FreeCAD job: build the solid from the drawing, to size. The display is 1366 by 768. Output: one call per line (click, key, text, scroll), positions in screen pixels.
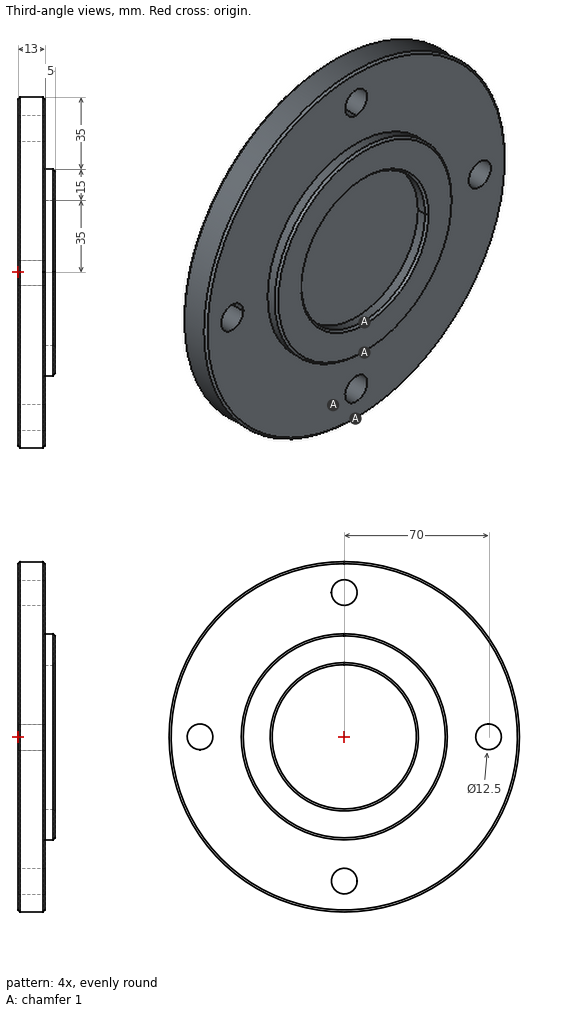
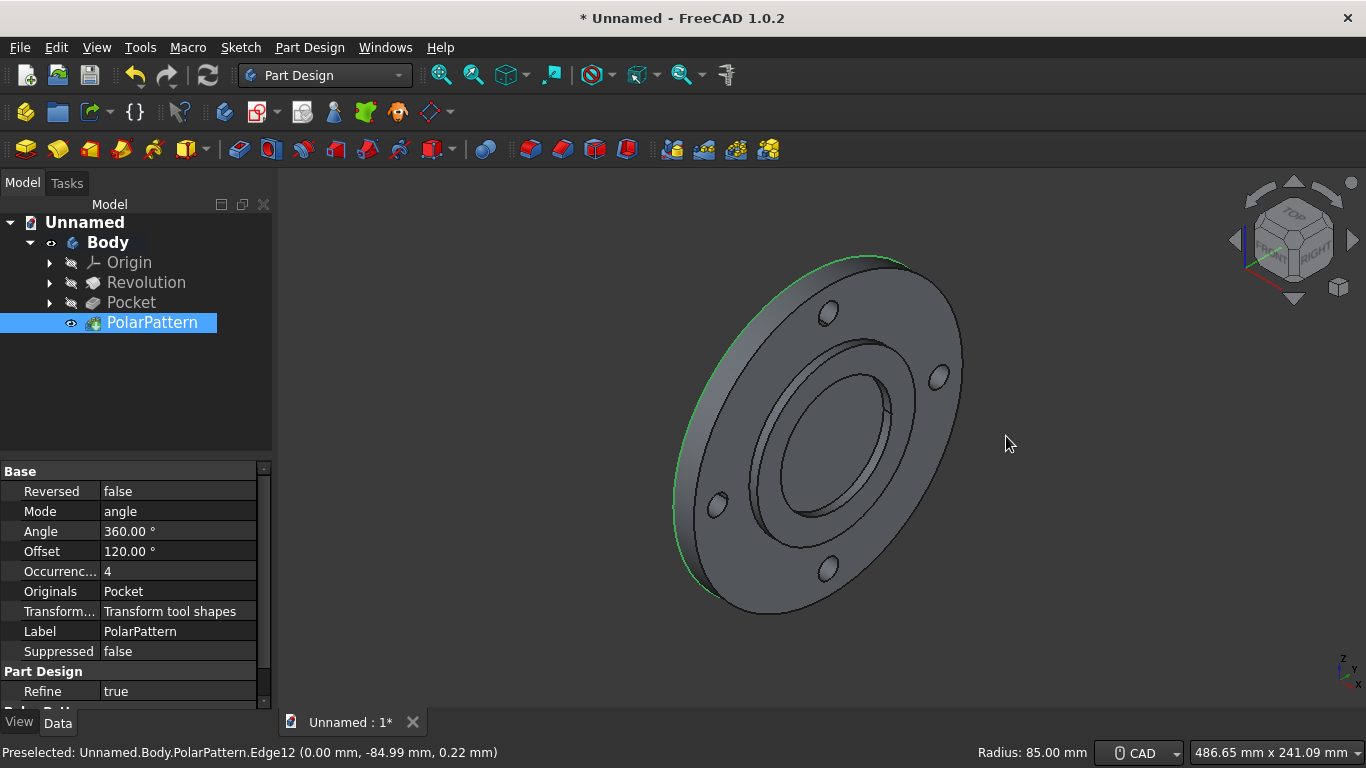
click(819, 515, ctrl)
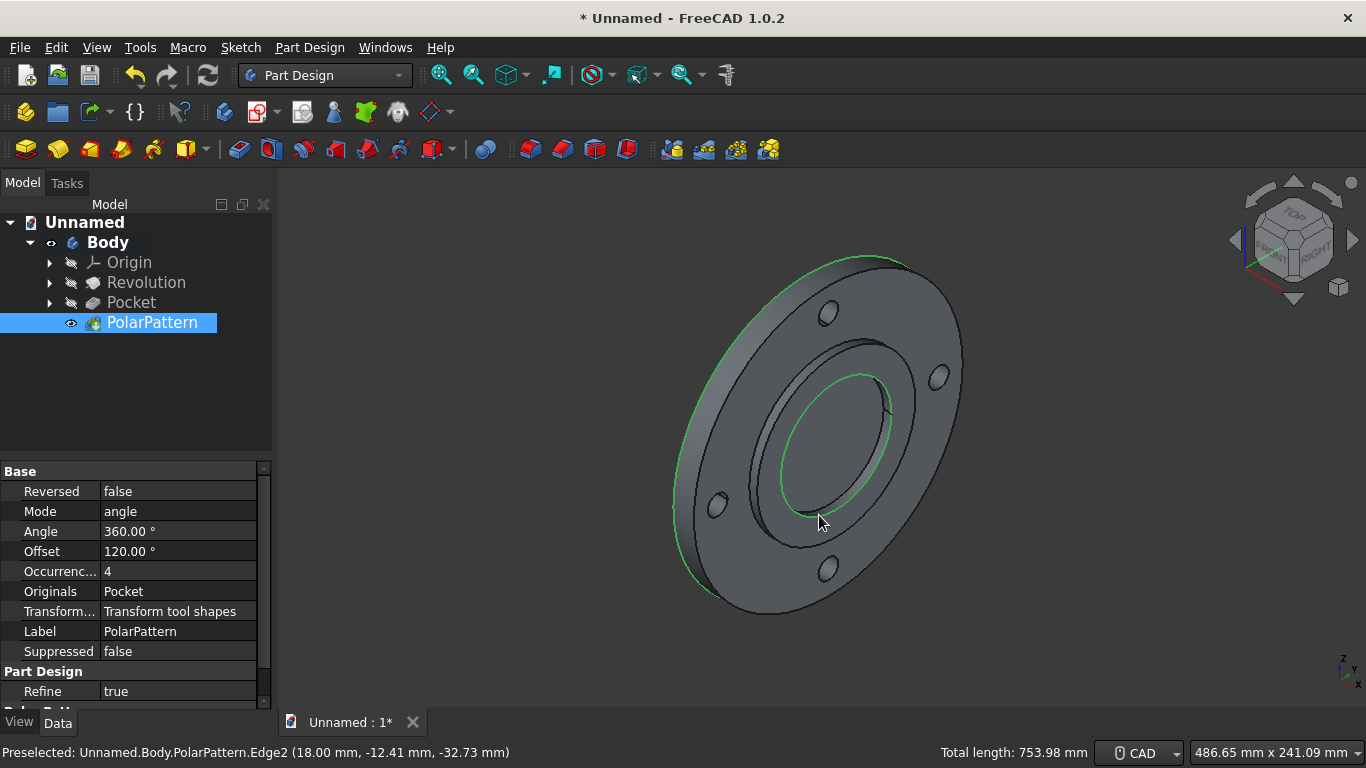
click(757, 490, ctrl)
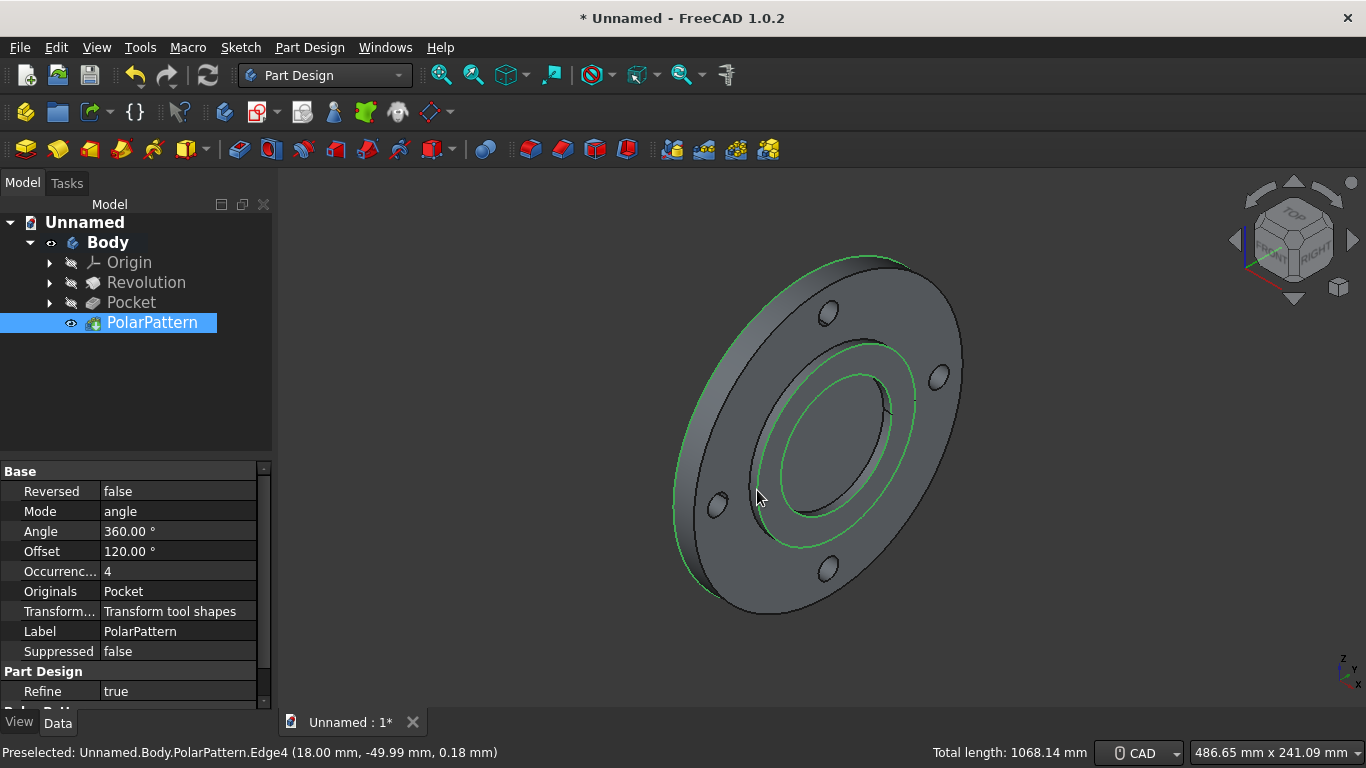
click(694, 518, ctrl)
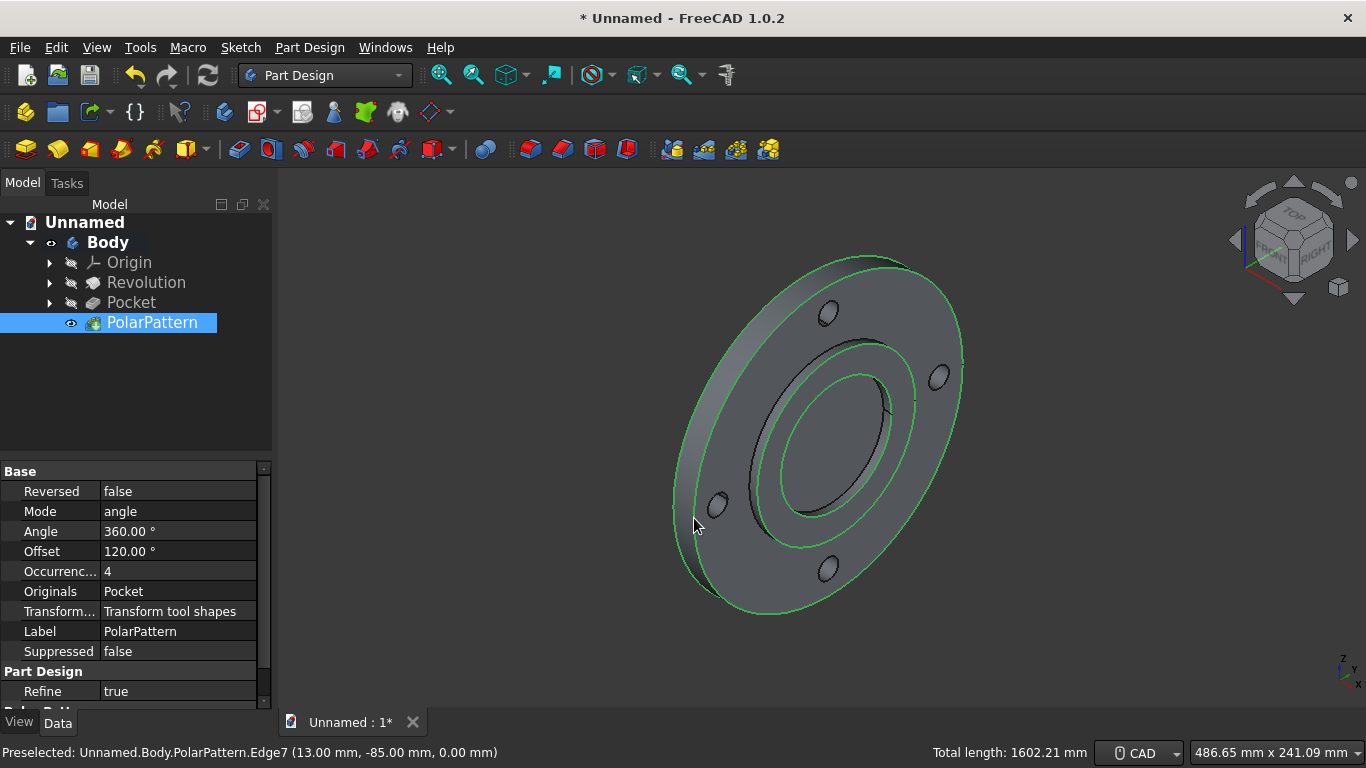
click(564, 150)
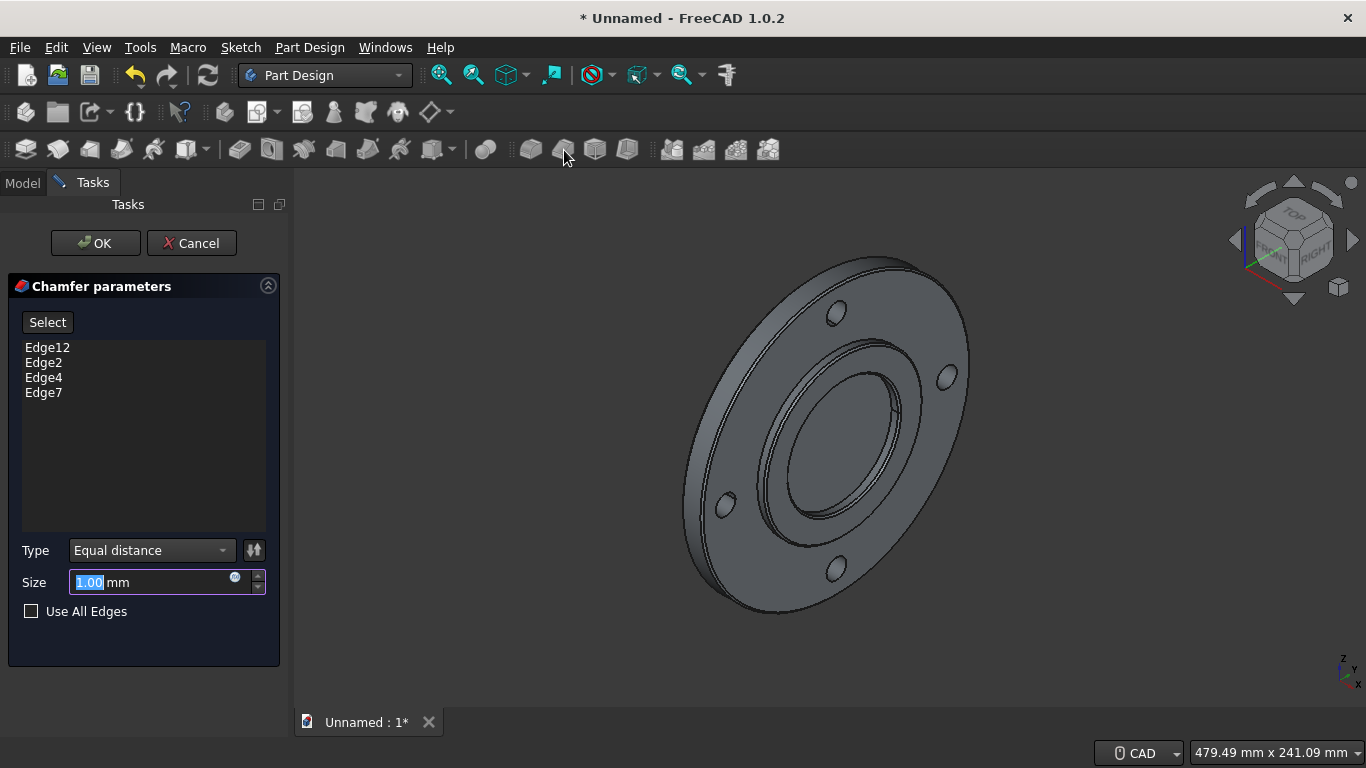
text(1)
key(Tab)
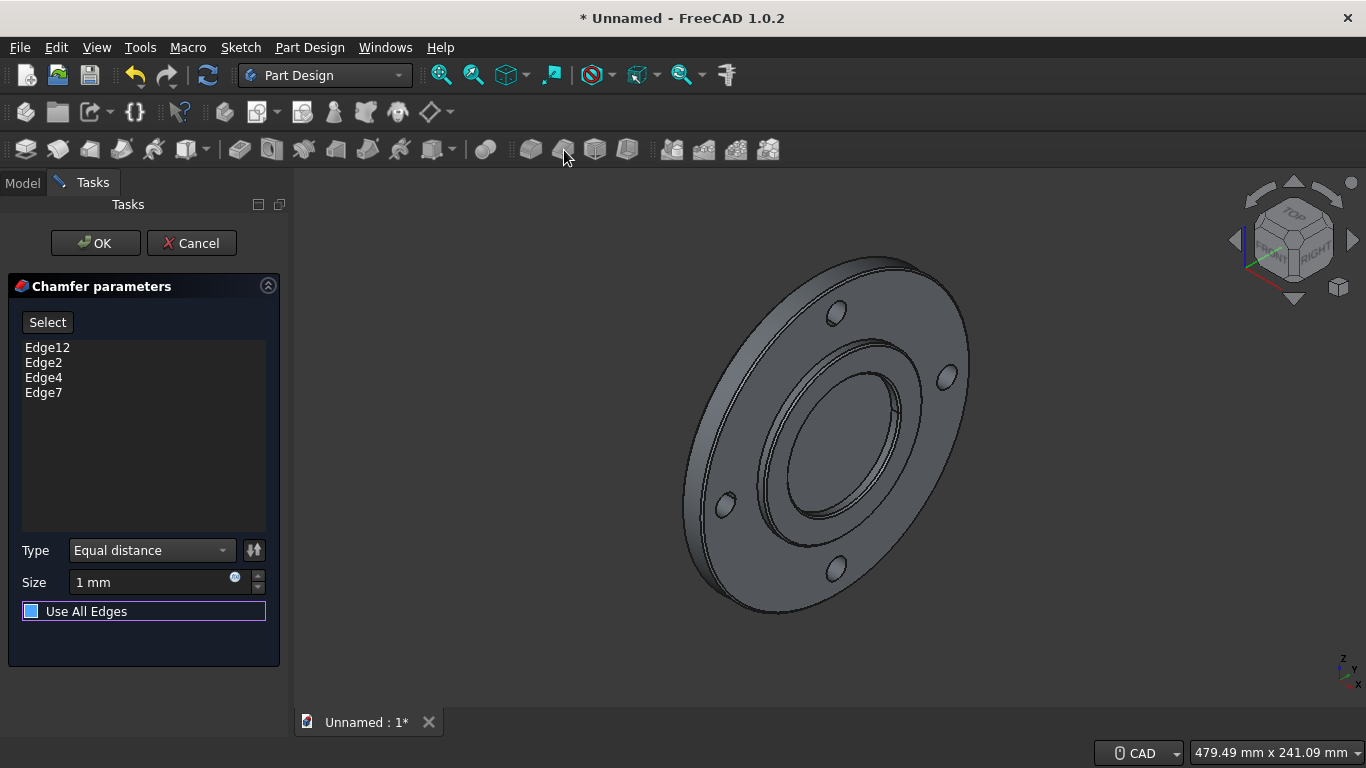
click(96, 243)